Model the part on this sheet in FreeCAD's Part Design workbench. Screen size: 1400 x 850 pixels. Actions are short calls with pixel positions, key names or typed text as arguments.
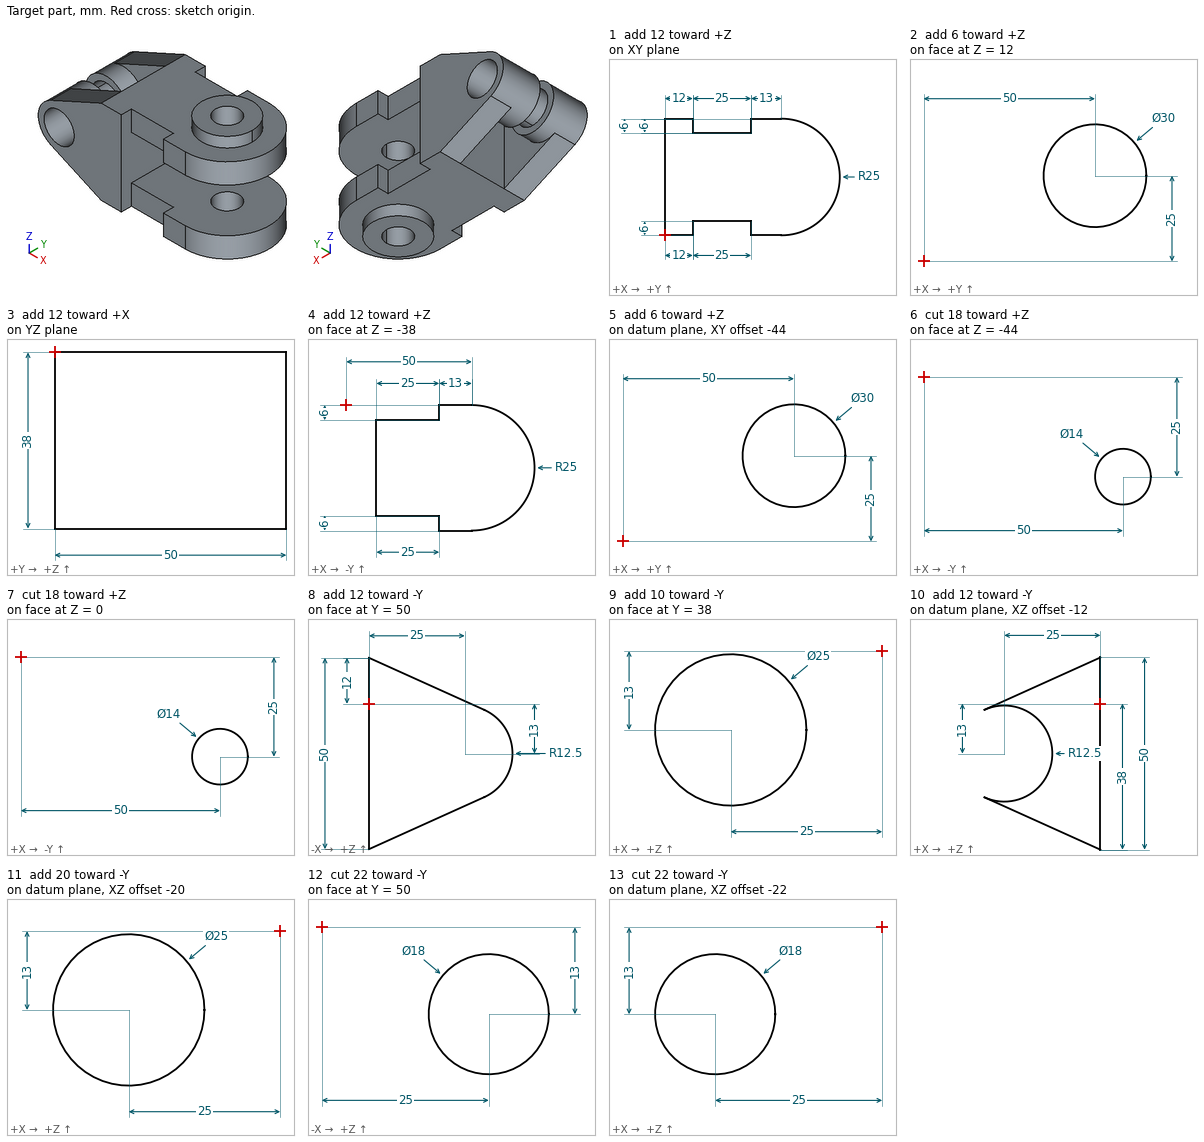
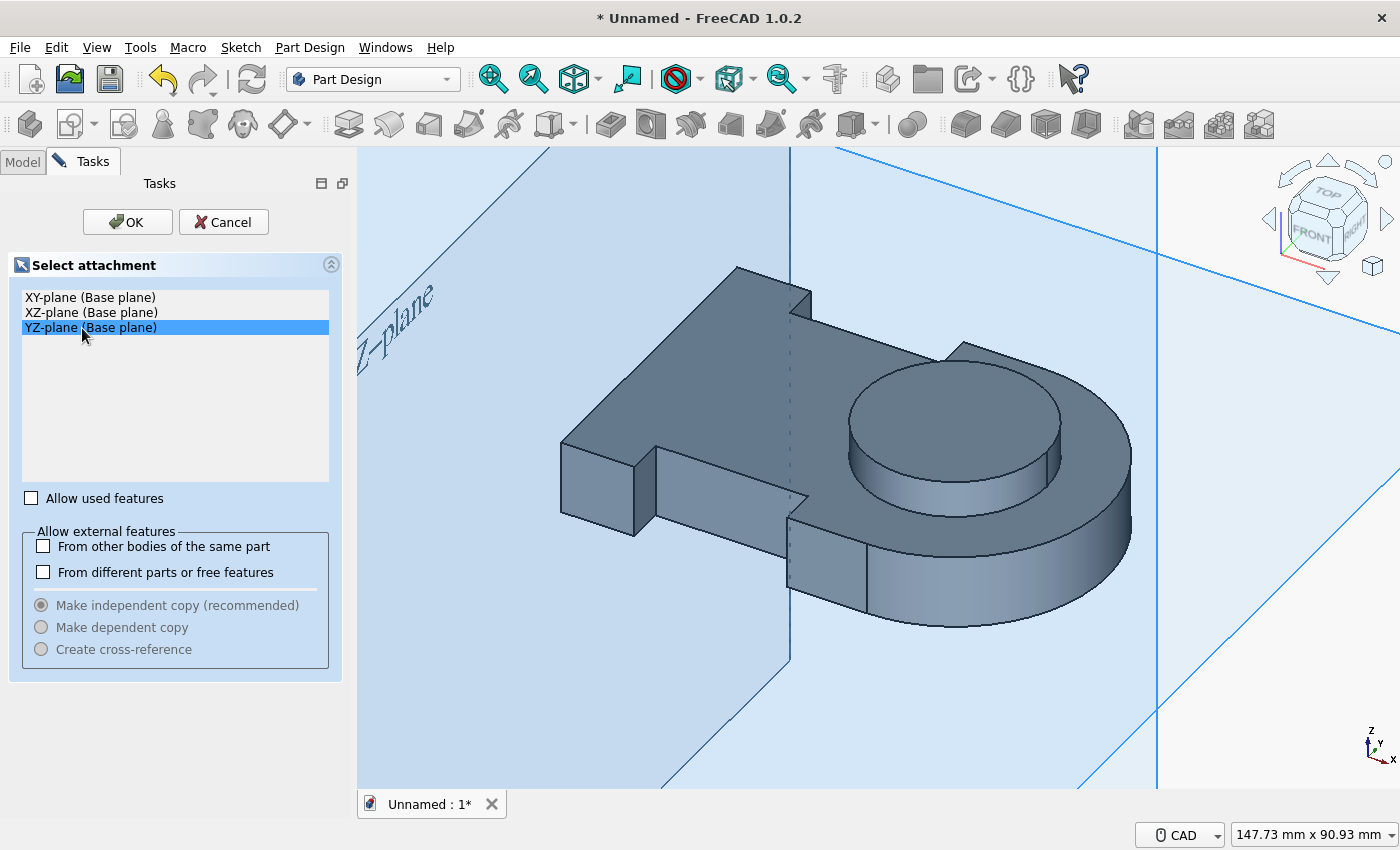
click(128, 222)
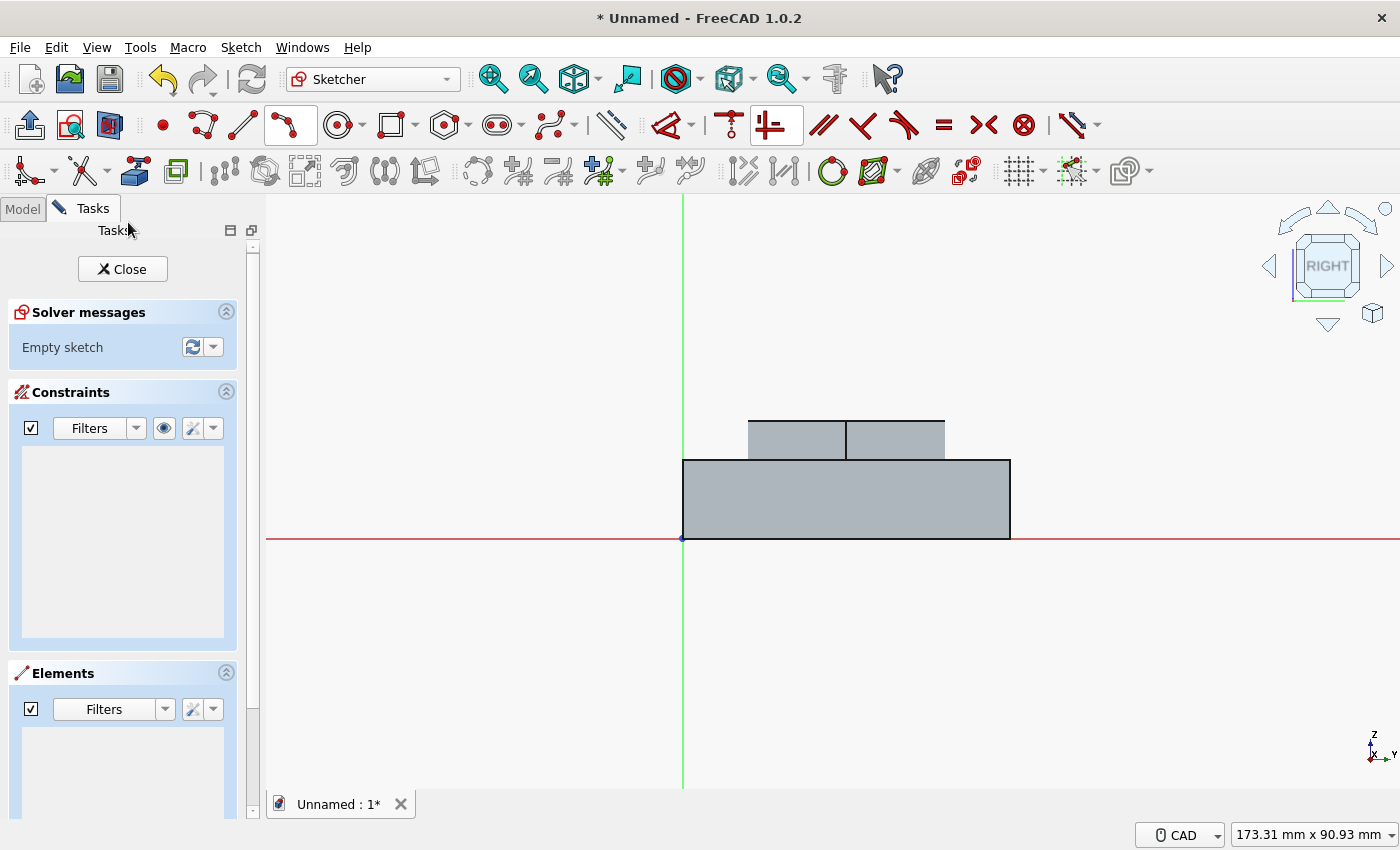
click(110, 126)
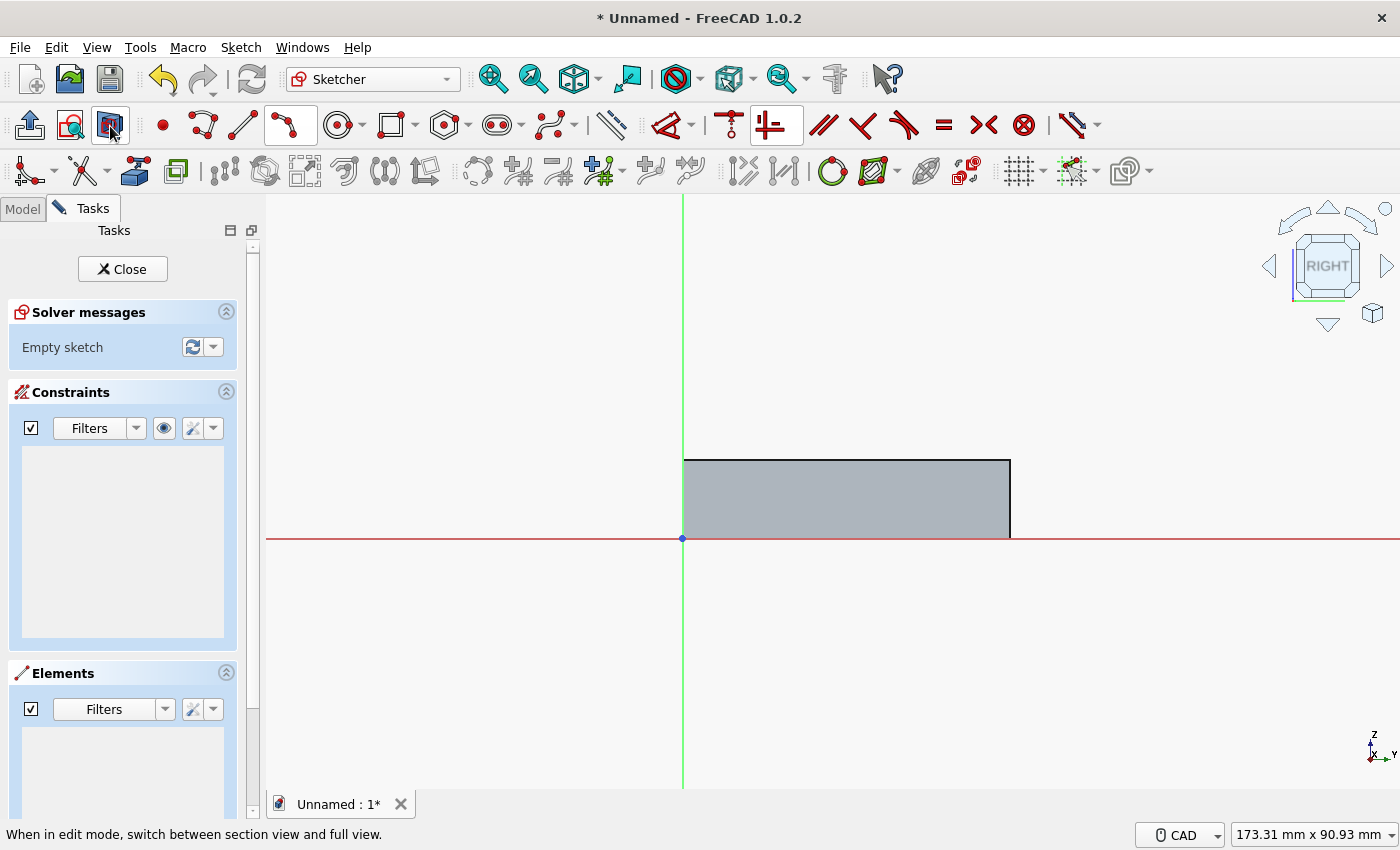
scroll(394, 222, down, 1)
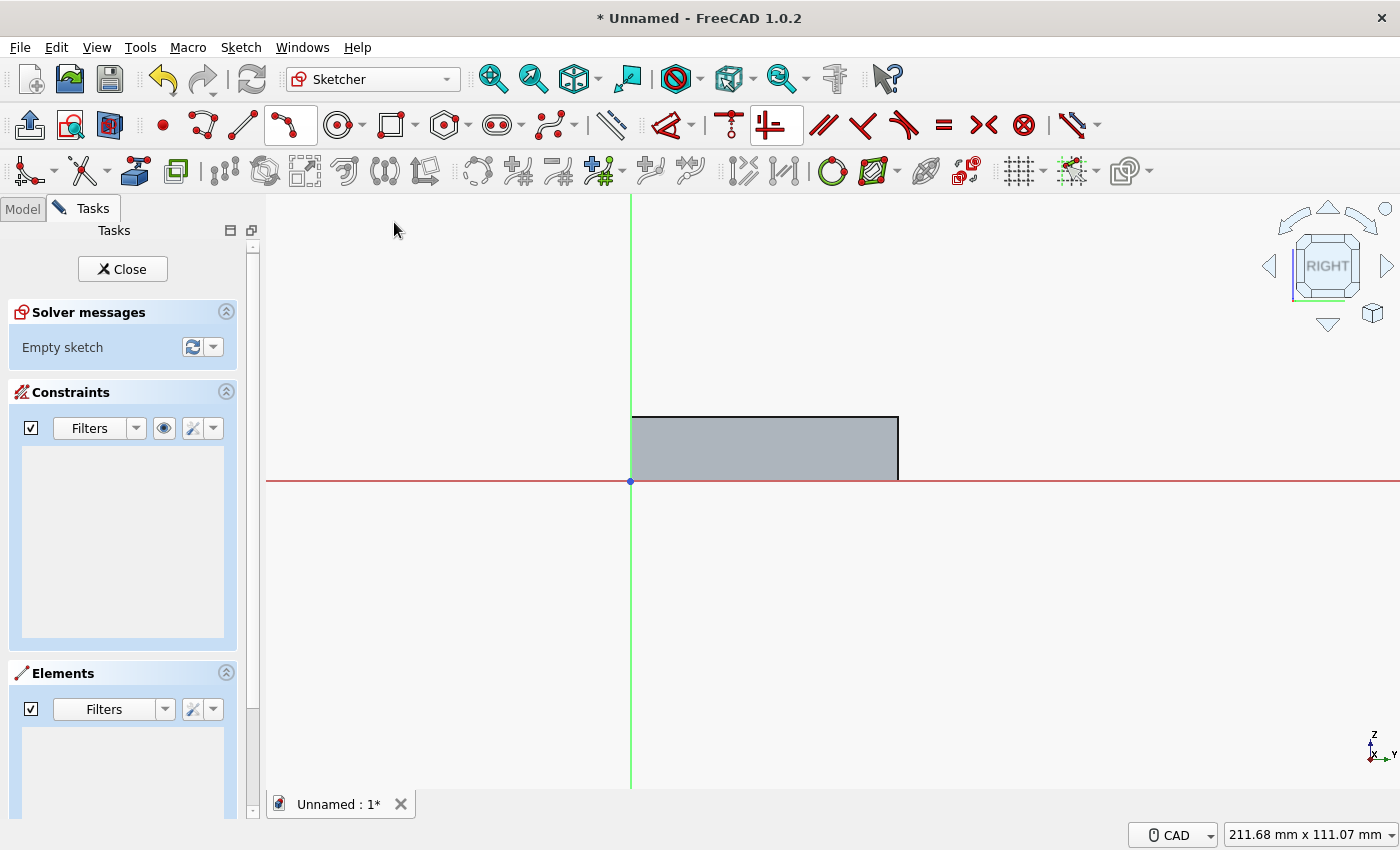
scroll(764, 695, up, 3)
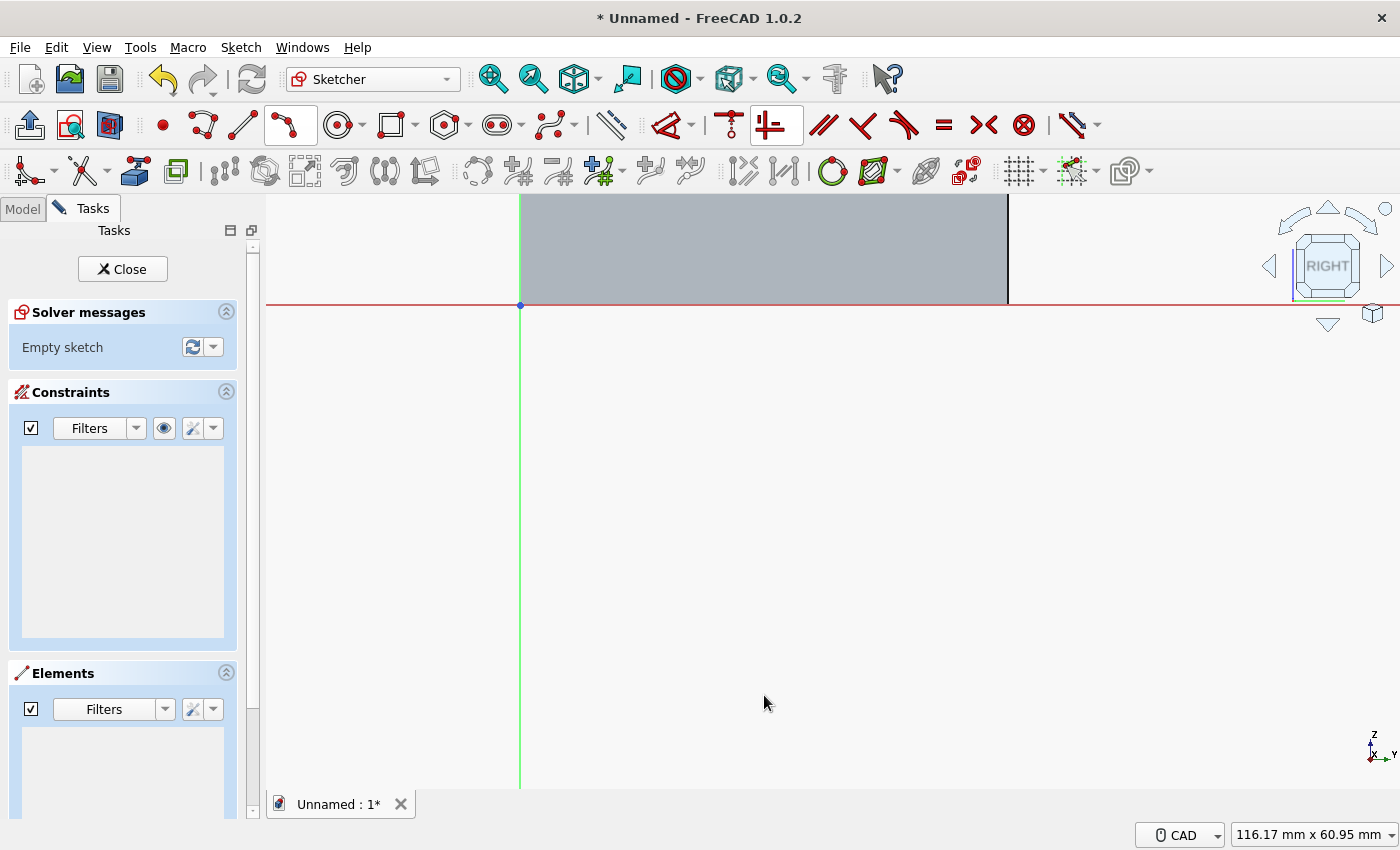
click(392, 126)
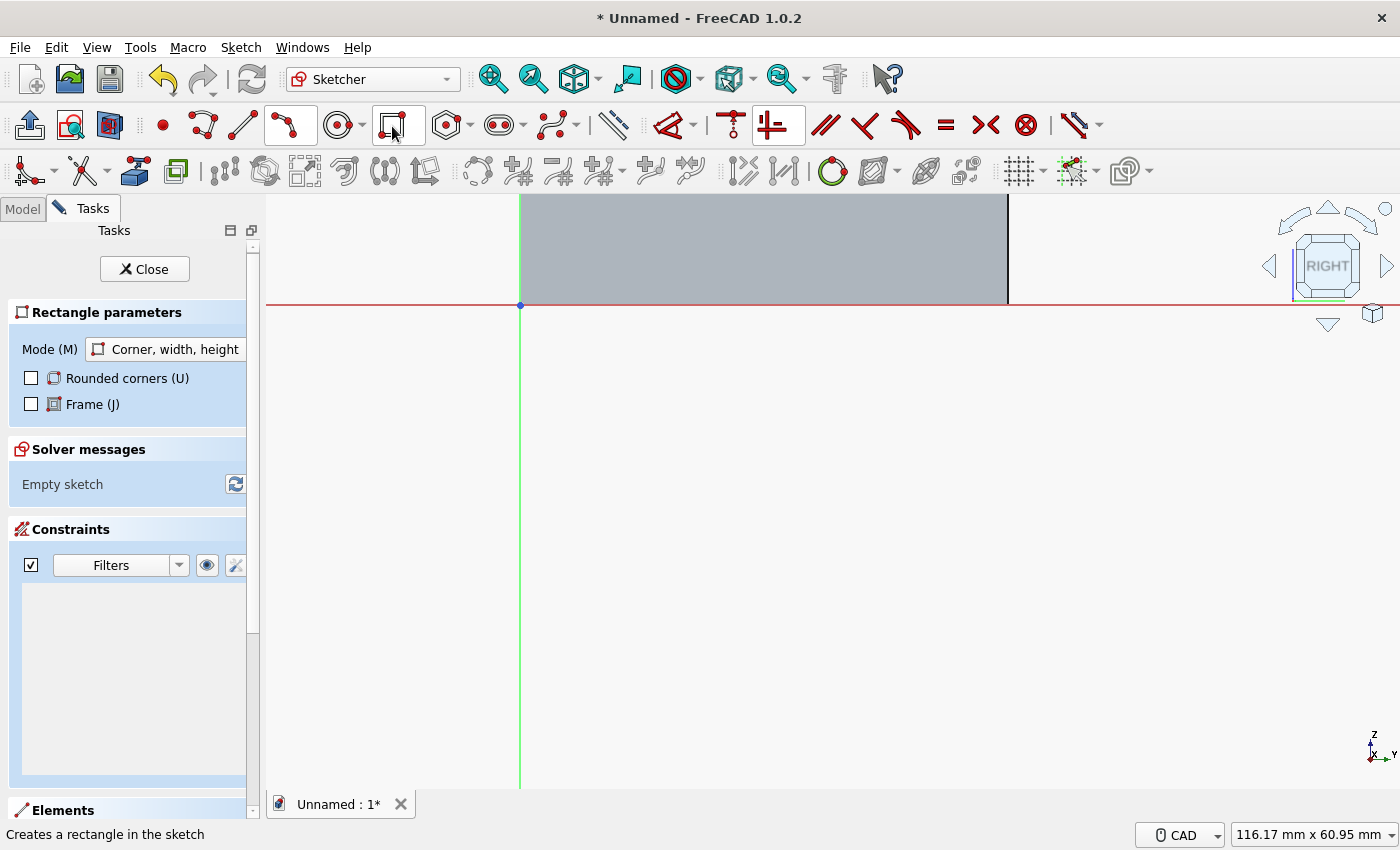
click(520, 305)
click(1008, 676)
key(Escape)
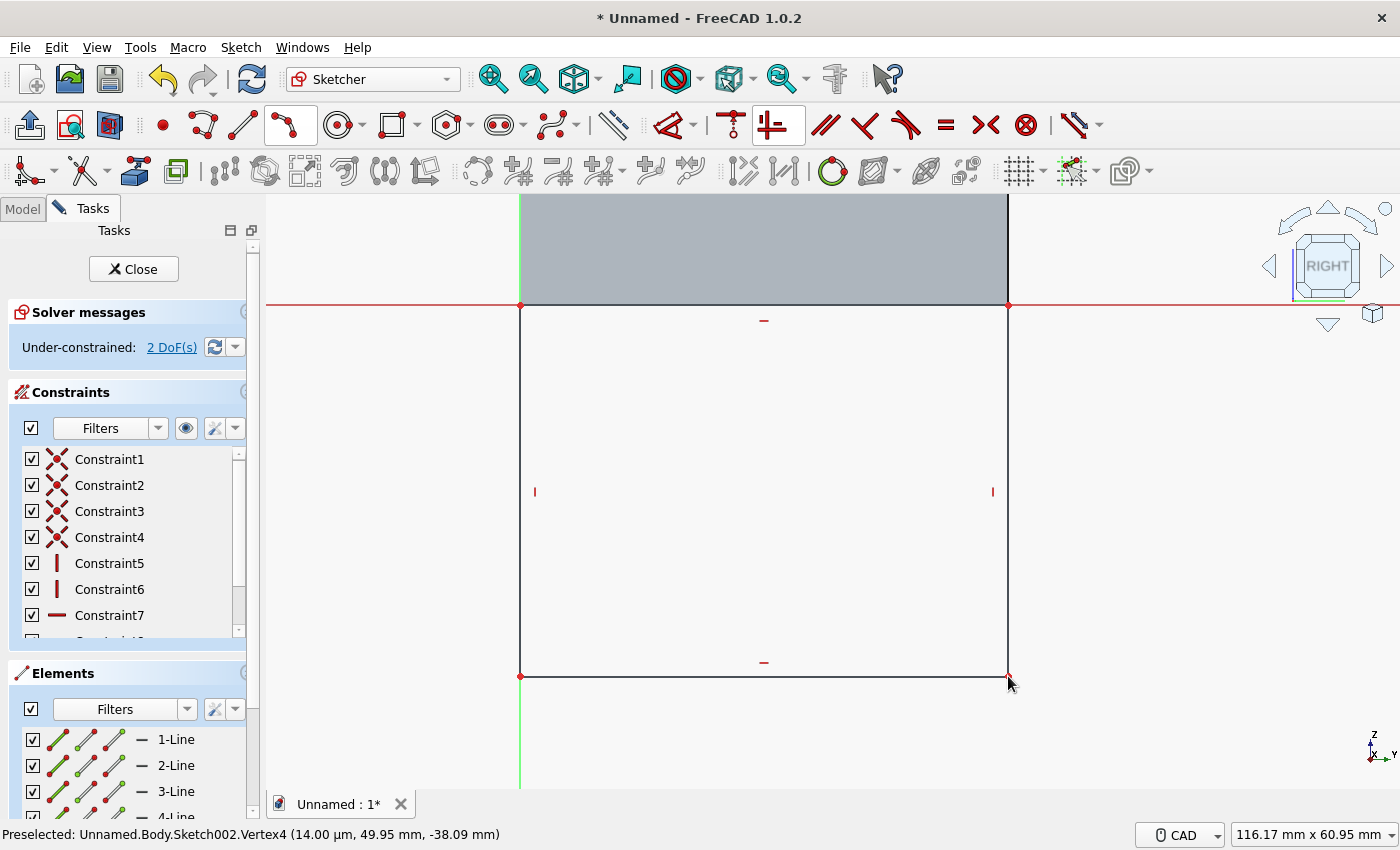
click(668, 126)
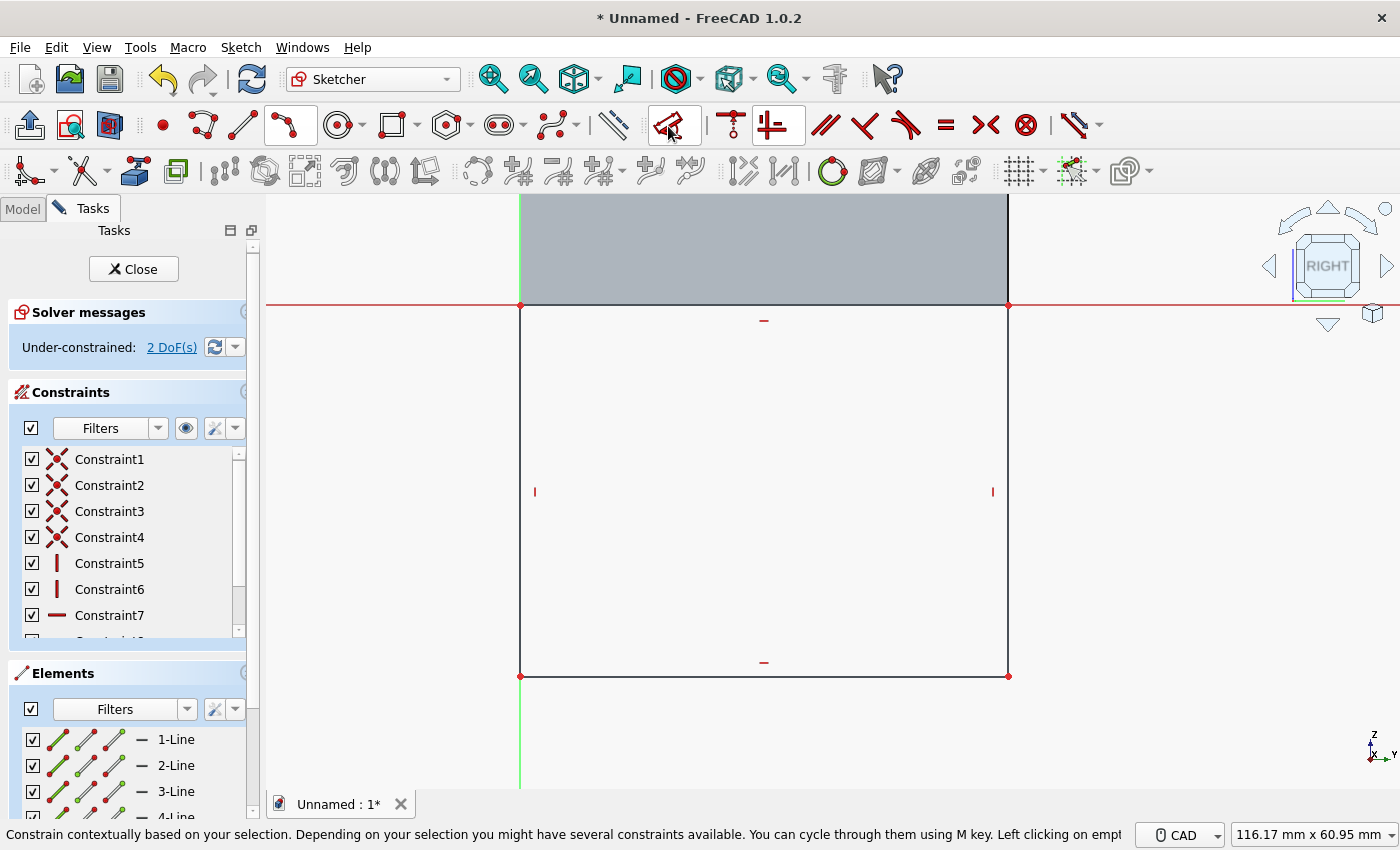
click(520, 417)
click(486, 491)